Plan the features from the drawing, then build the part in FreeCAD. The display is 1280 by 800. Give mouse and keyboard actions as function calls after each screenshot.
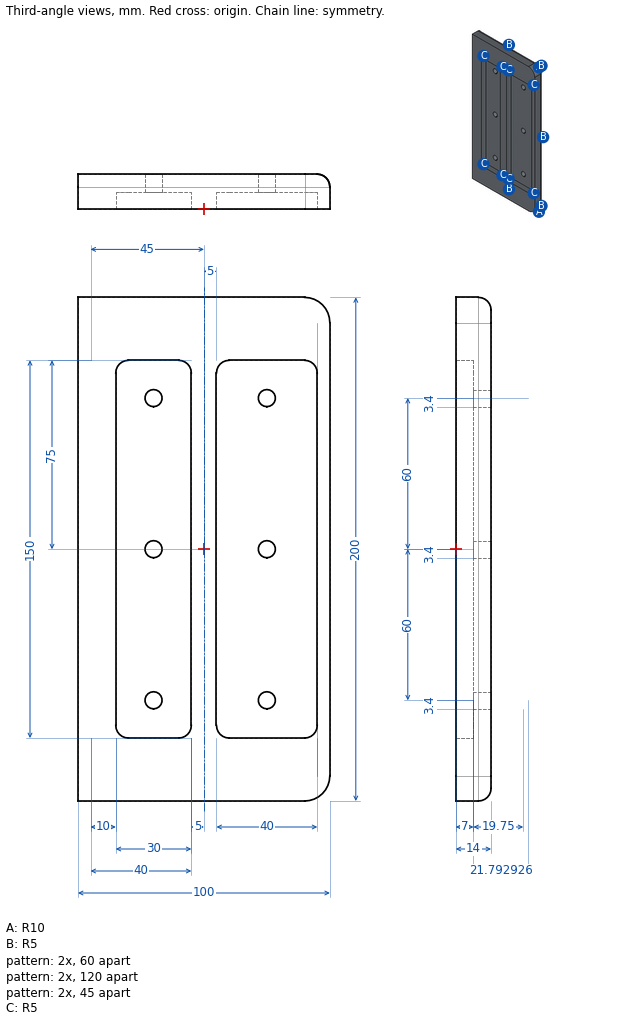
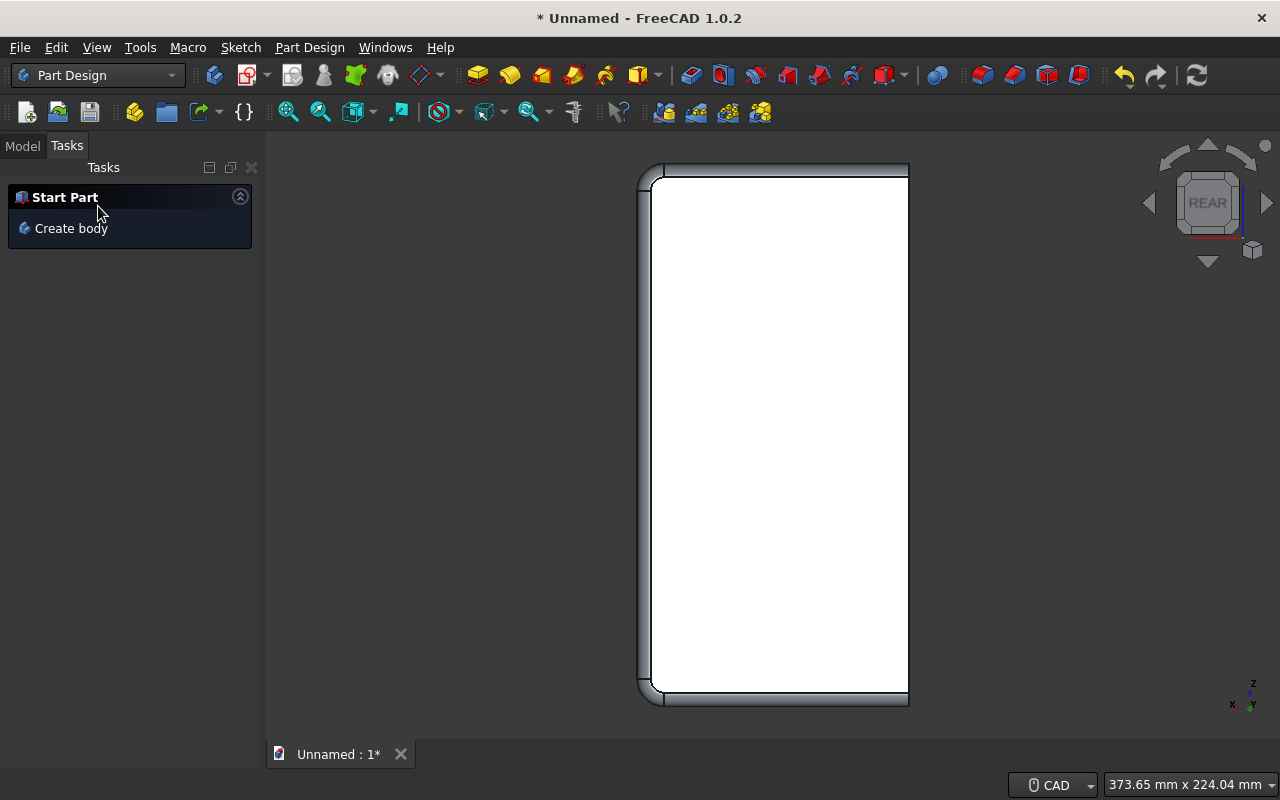
click(248, 76)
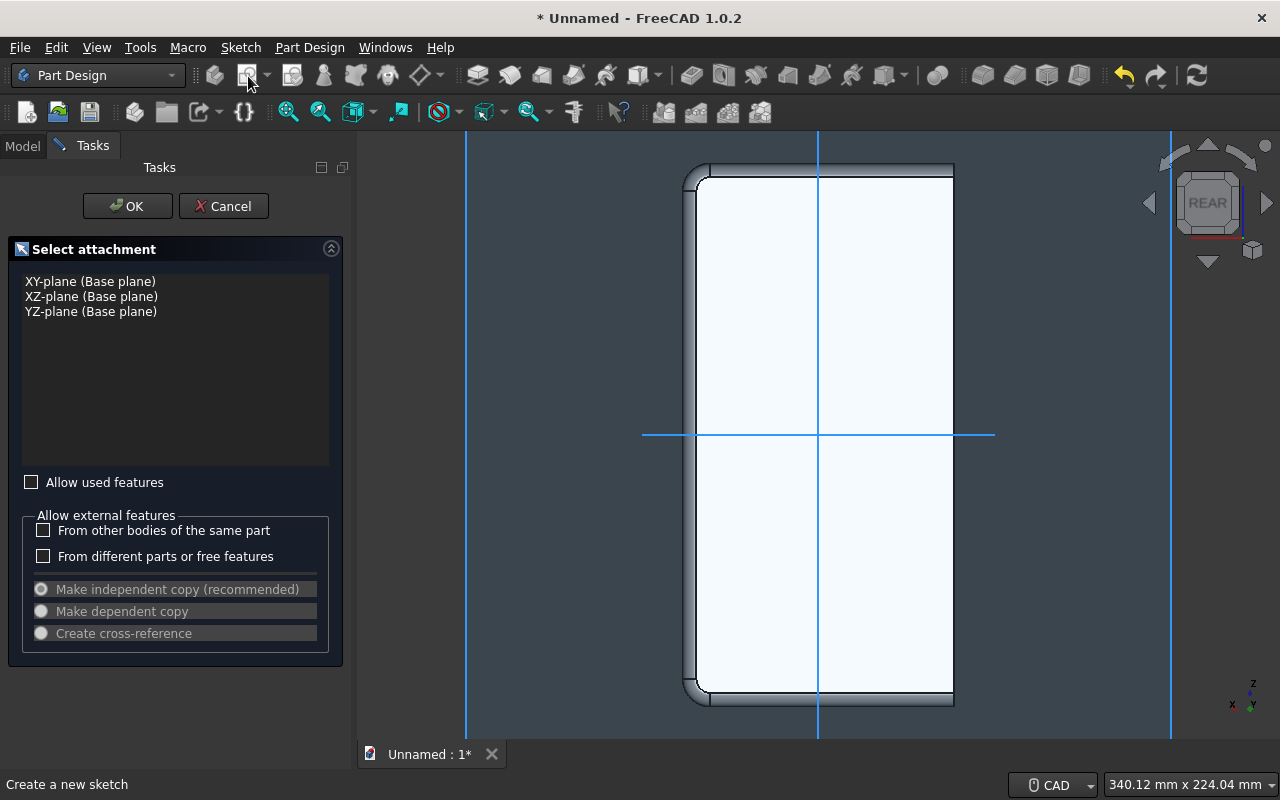
click(82, 296)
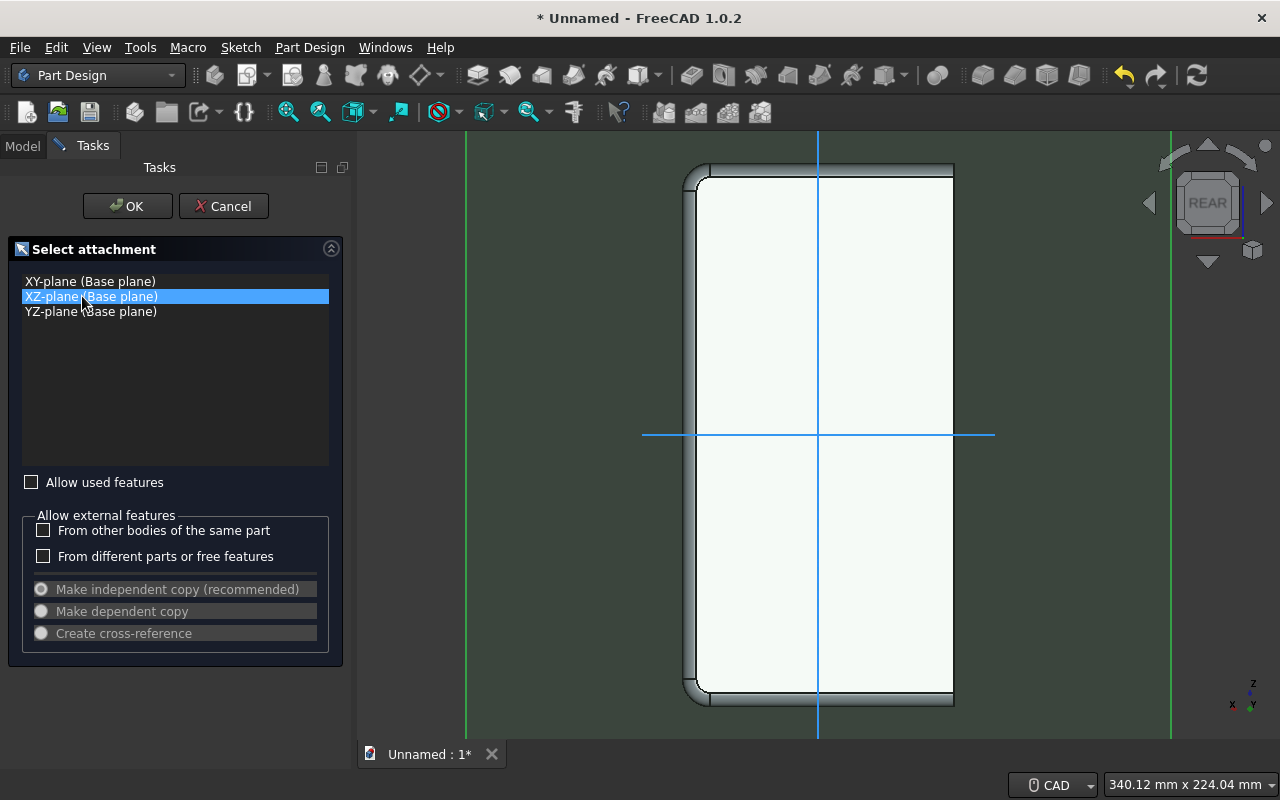
click(128, 206)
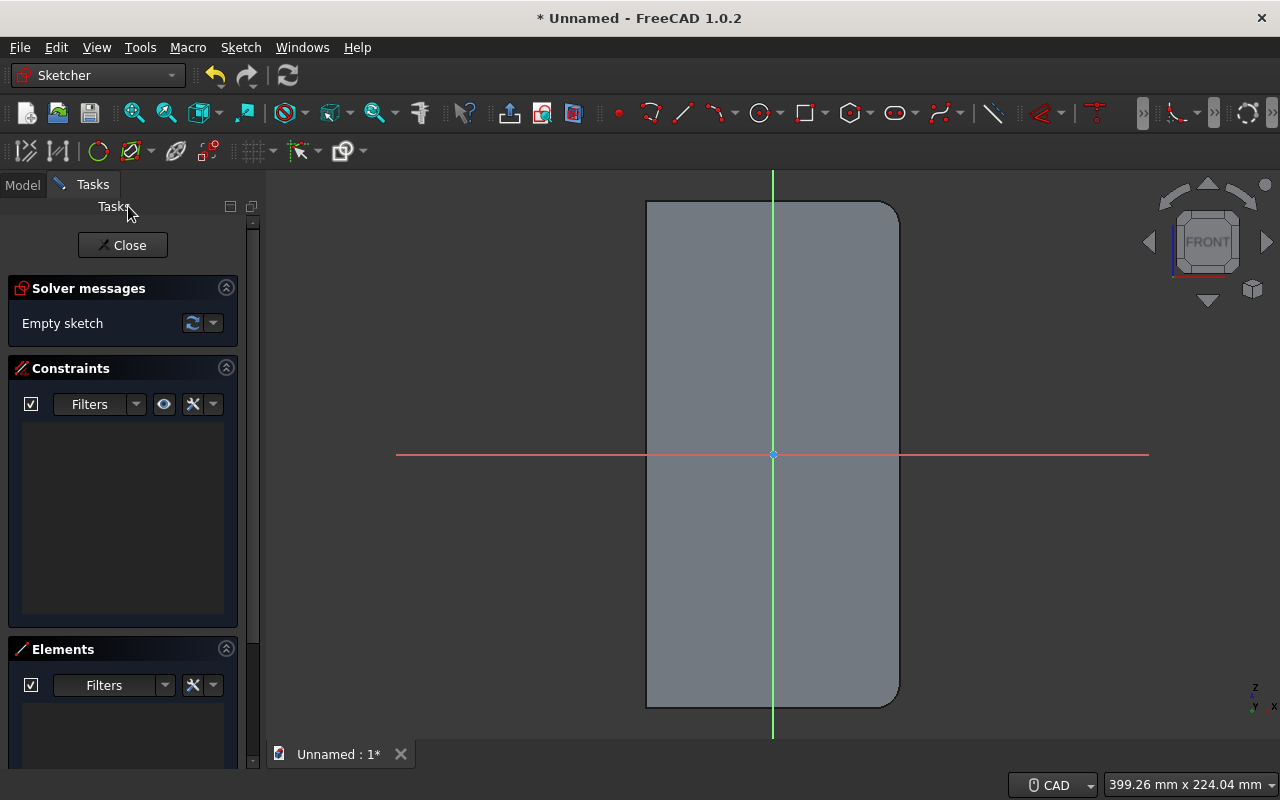
click(806, 114)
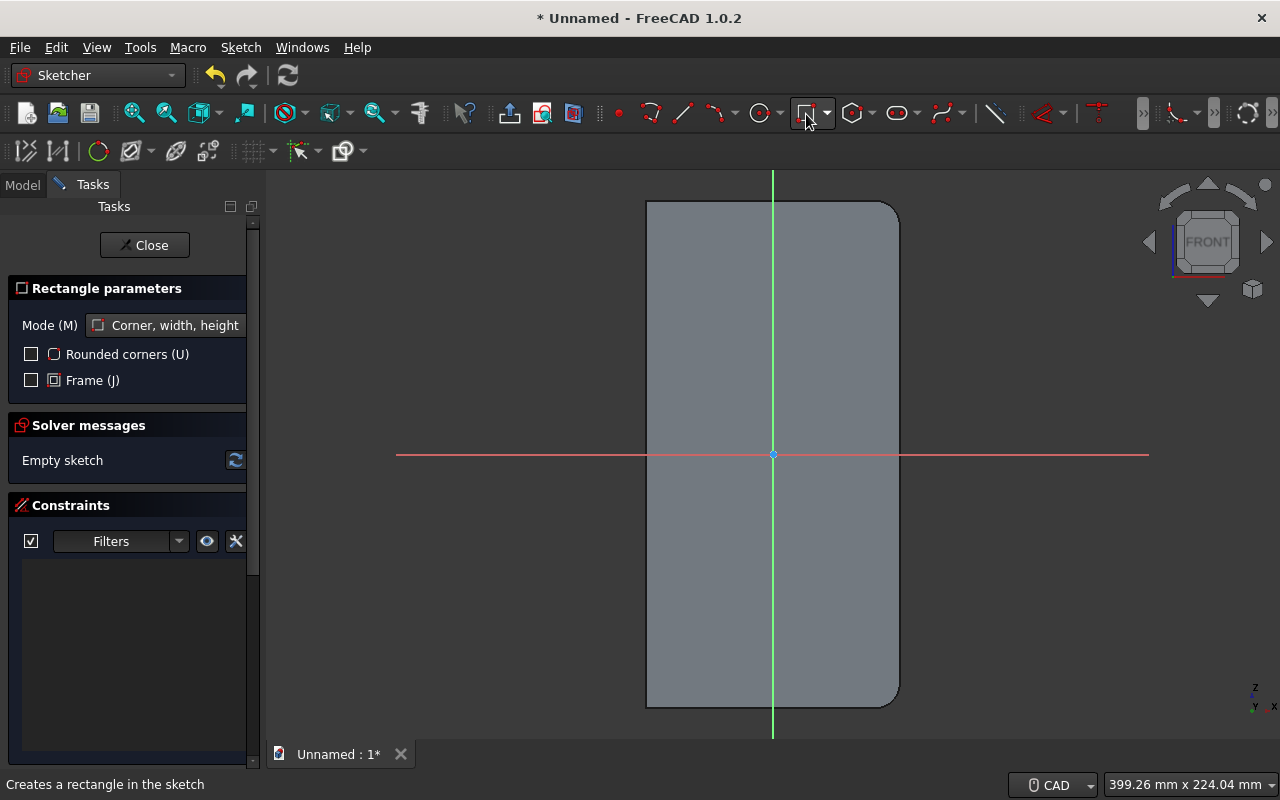
click(659, 264)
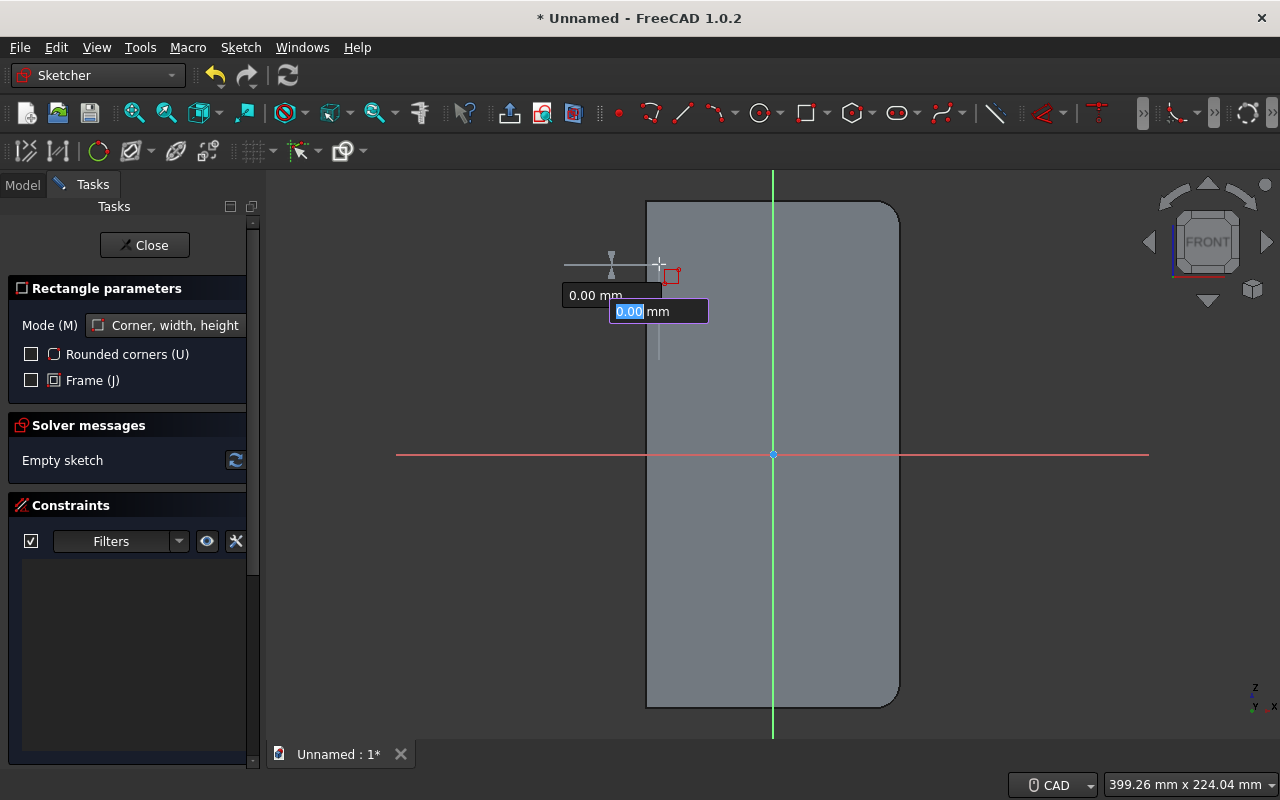
scroll(760, 645, up, 2)
move(760, 645)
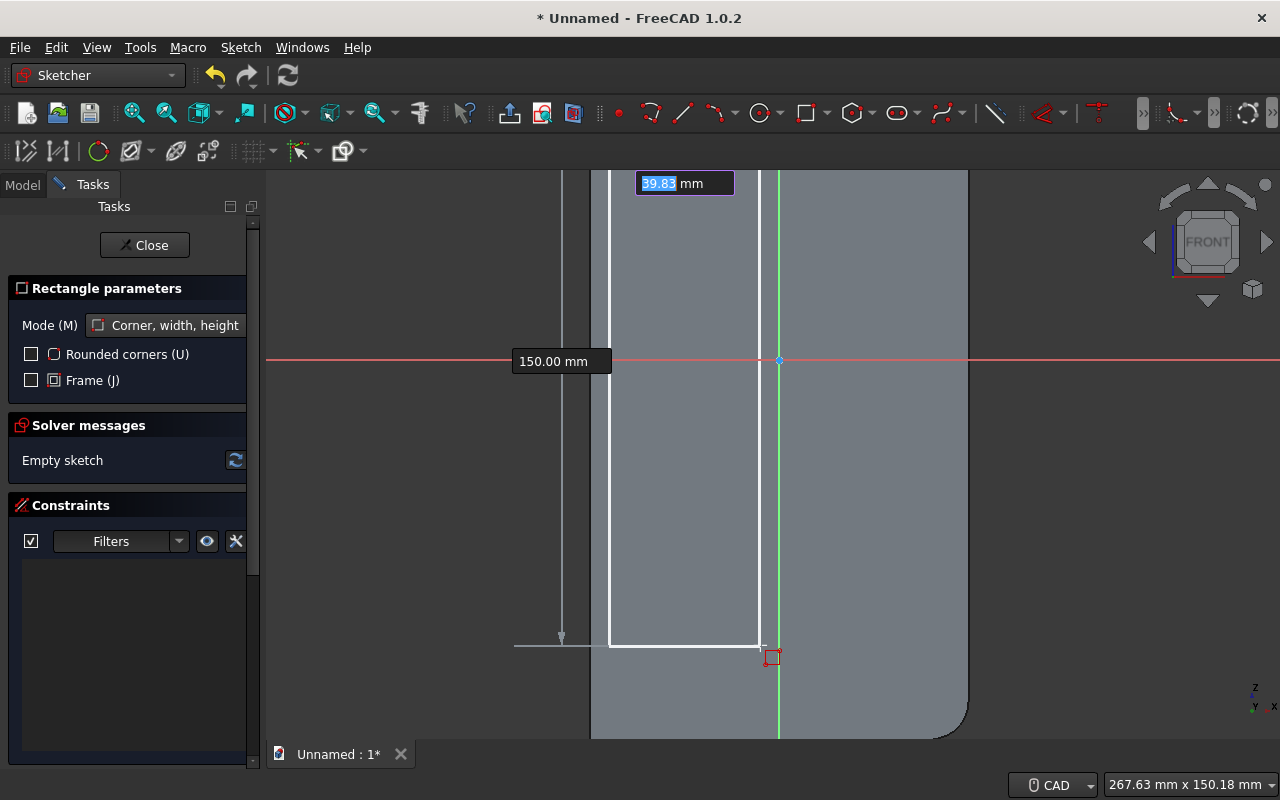
text(40)
key(Tab)
text(150)
key(Return)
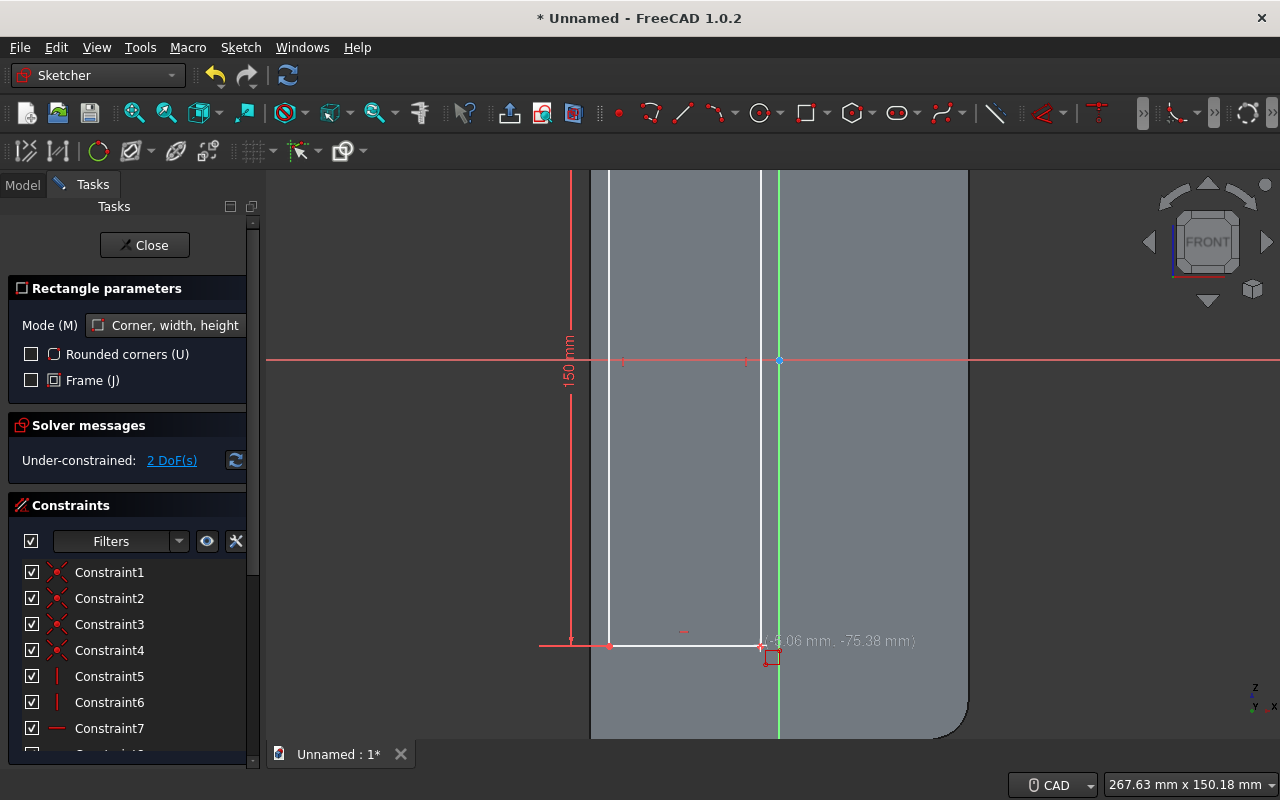
scroll(553, 646, down, 2)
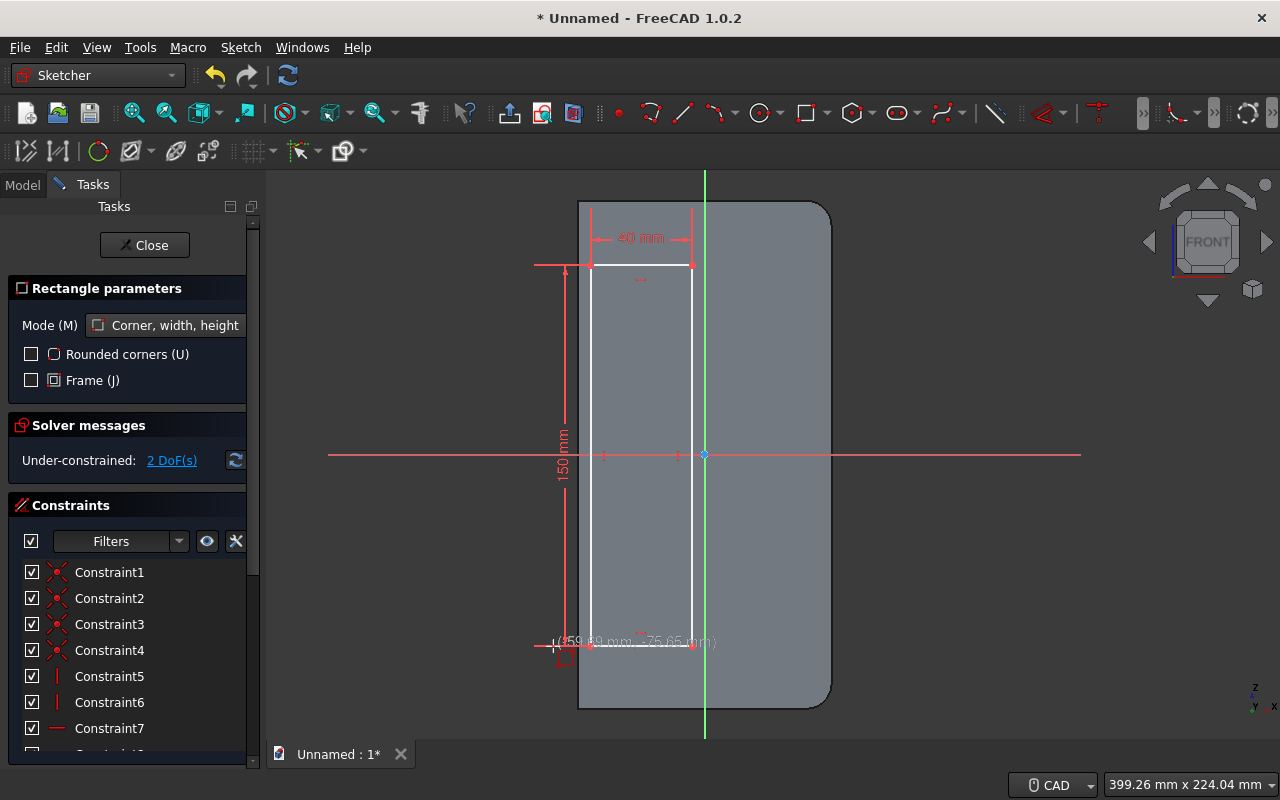
scroll(717, 264, up, 2)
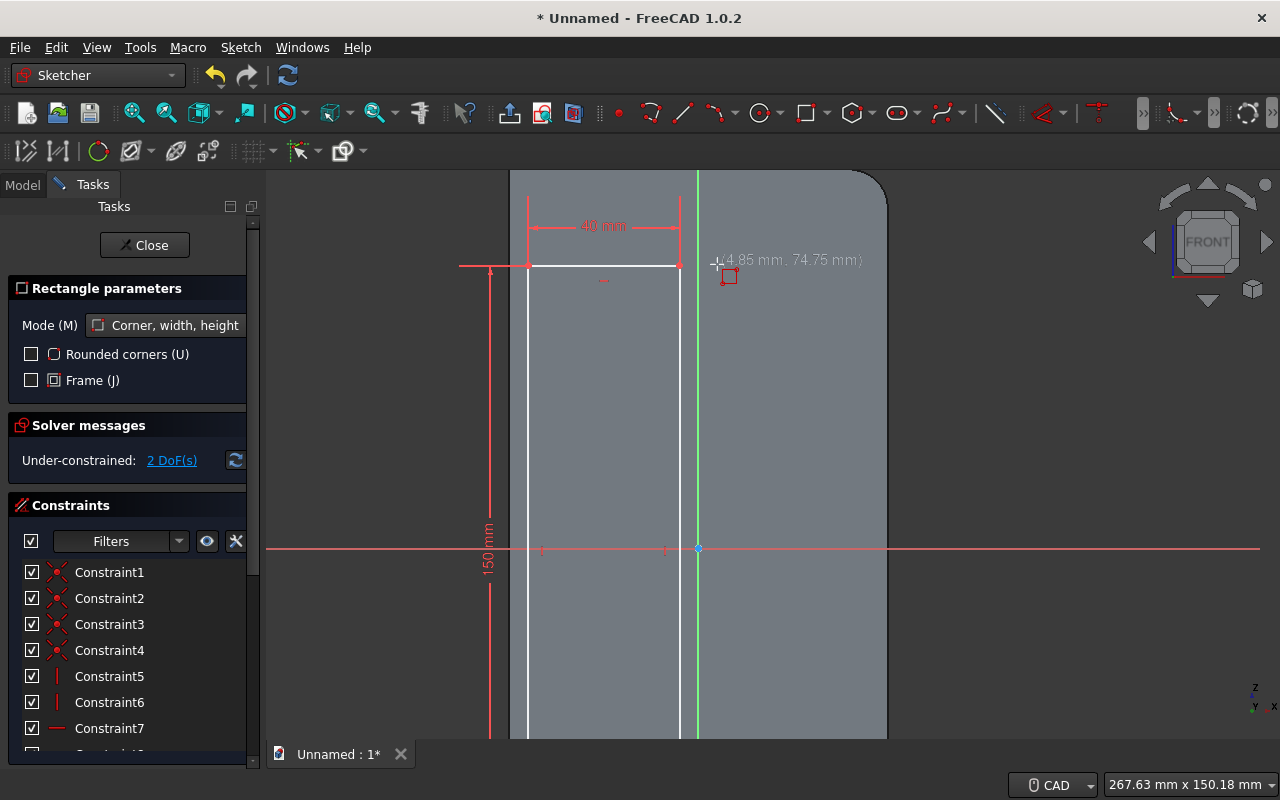
click(717, 264)